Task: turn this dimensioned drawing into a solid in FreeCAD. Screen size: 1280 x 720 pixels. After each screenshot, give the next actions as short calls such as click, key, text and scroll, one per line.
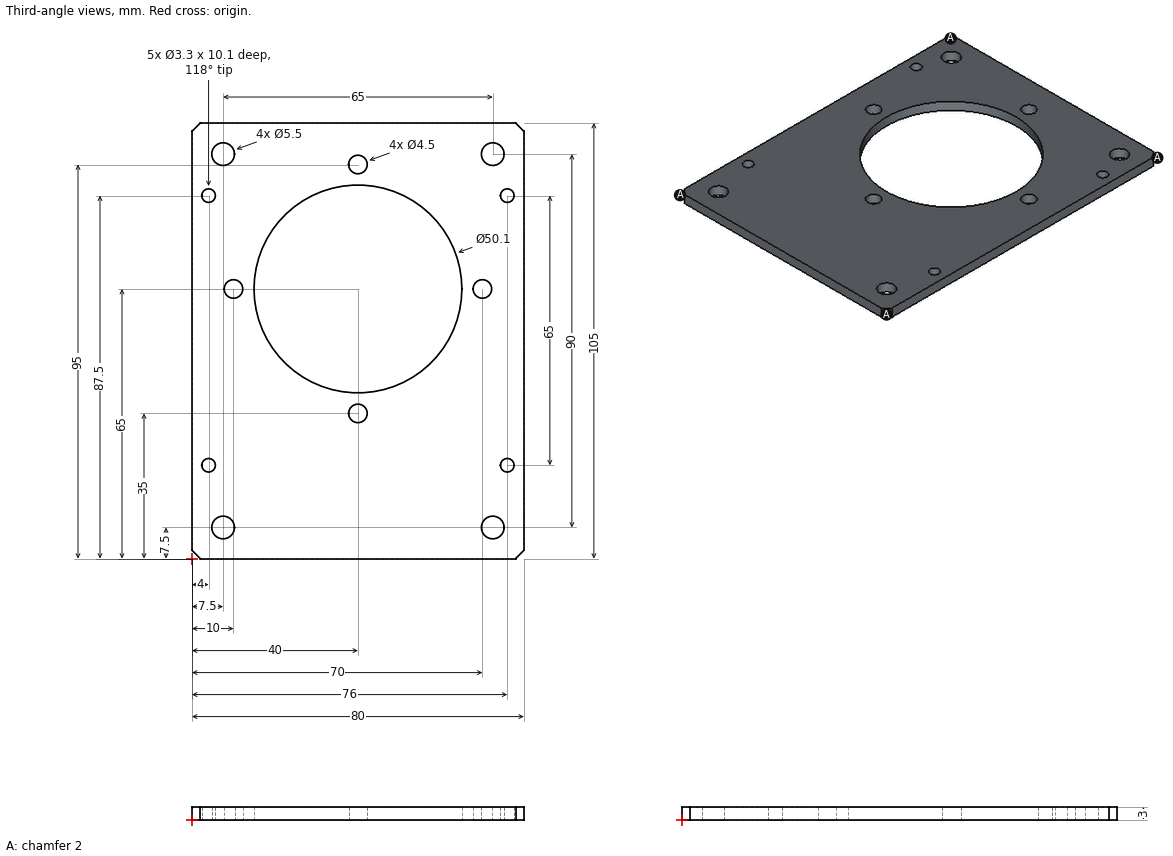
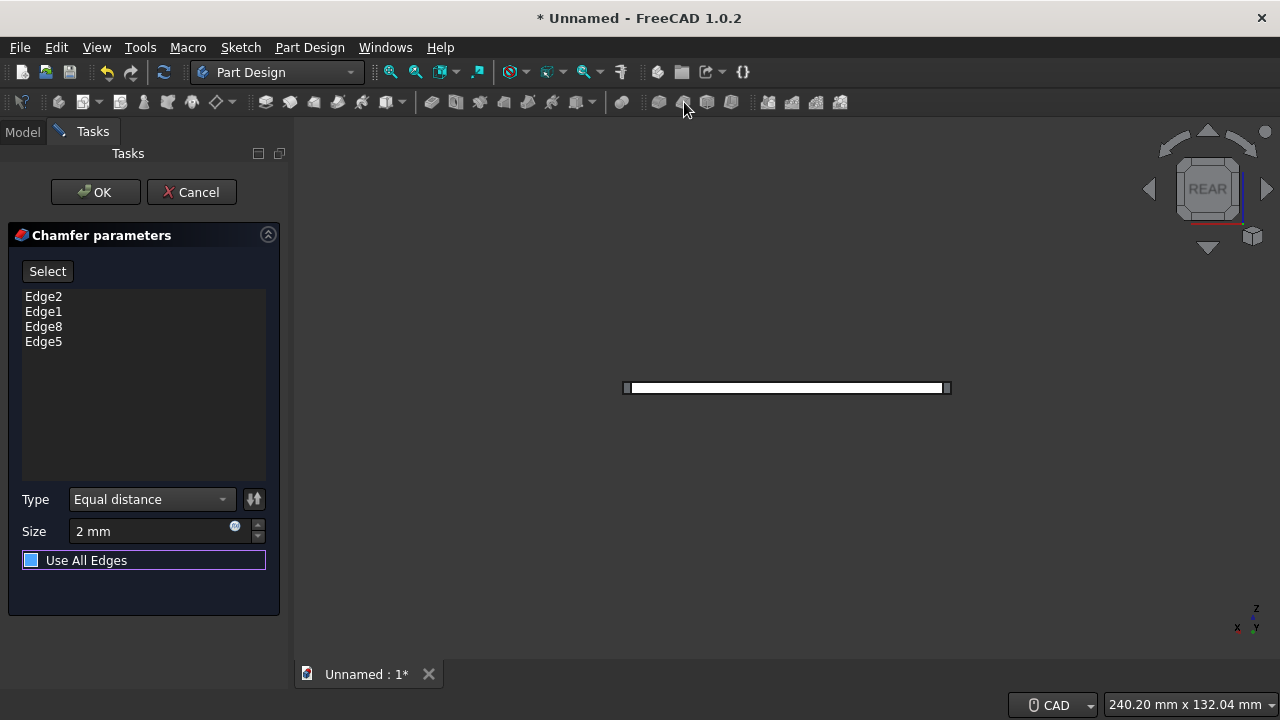
click(96, 192)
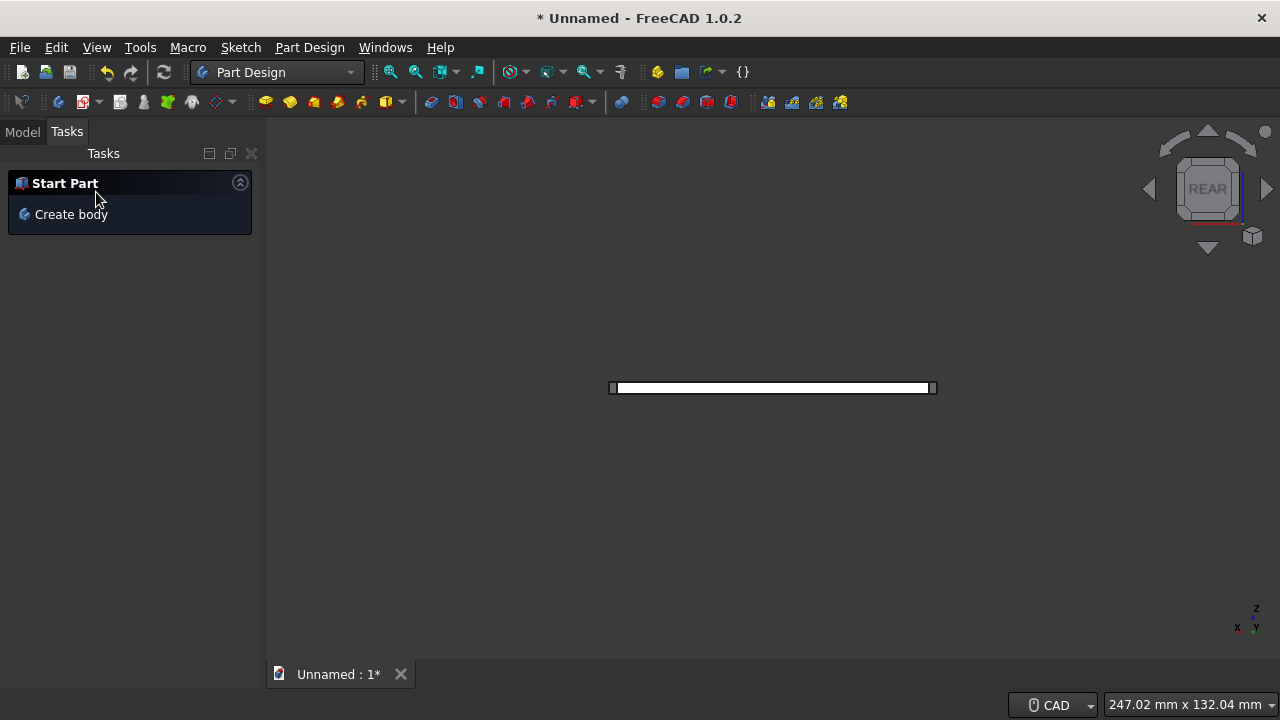
click(392, 72)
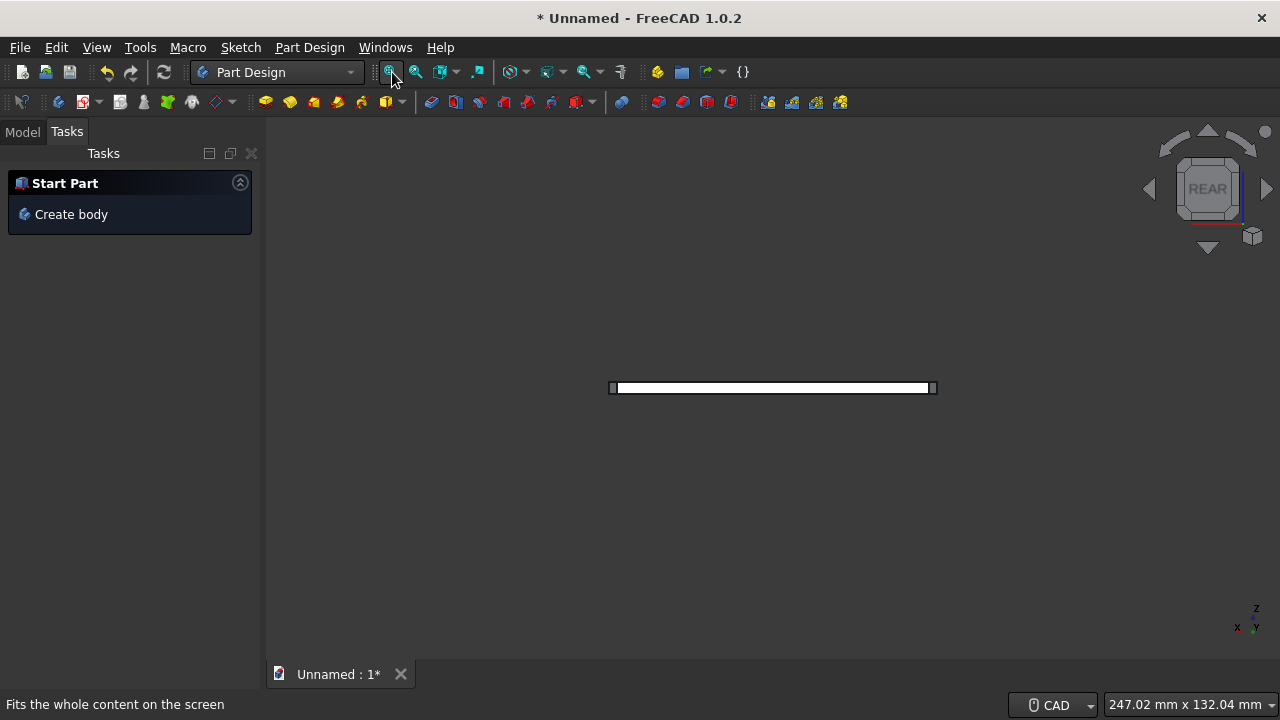
key(0)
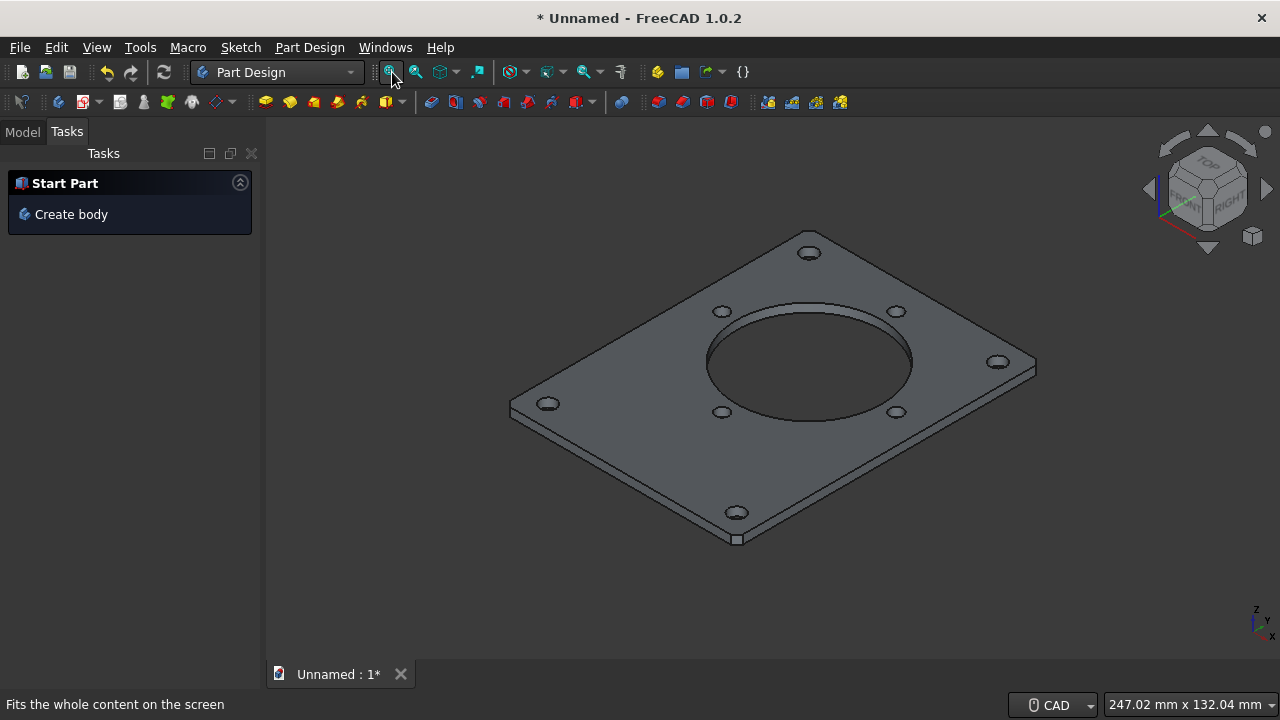
click(752, 471)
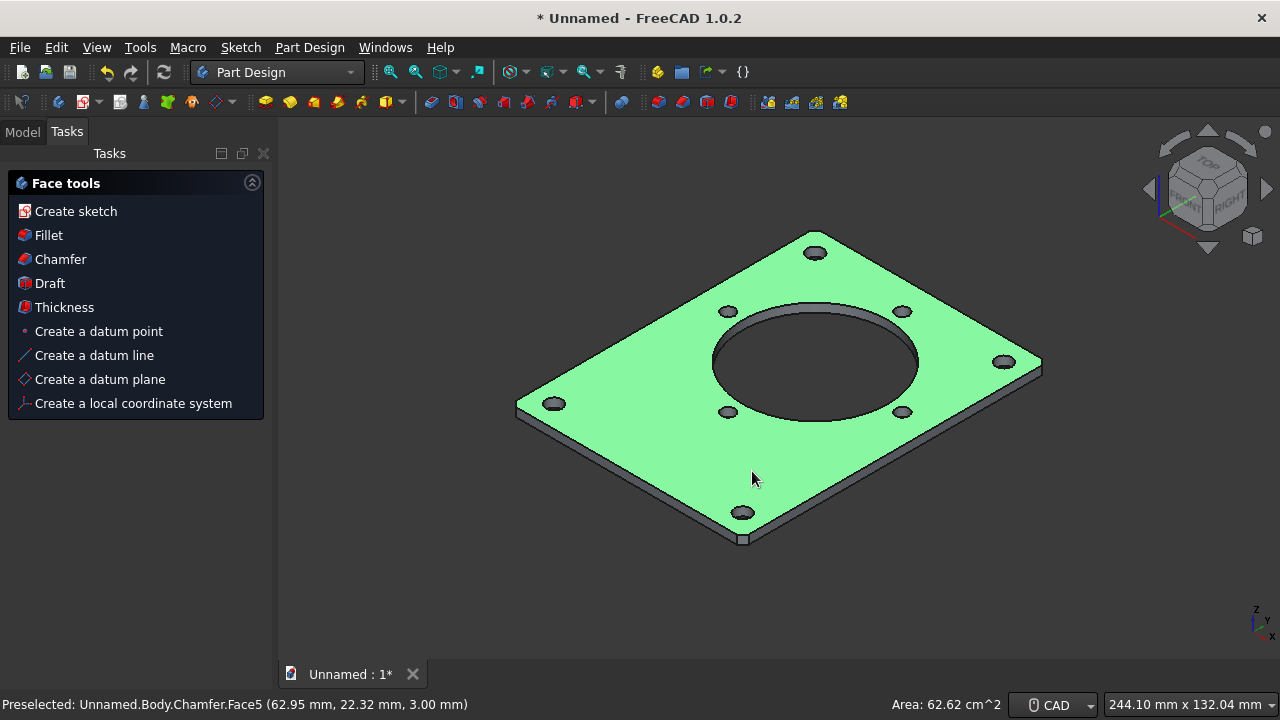
click(84, 102)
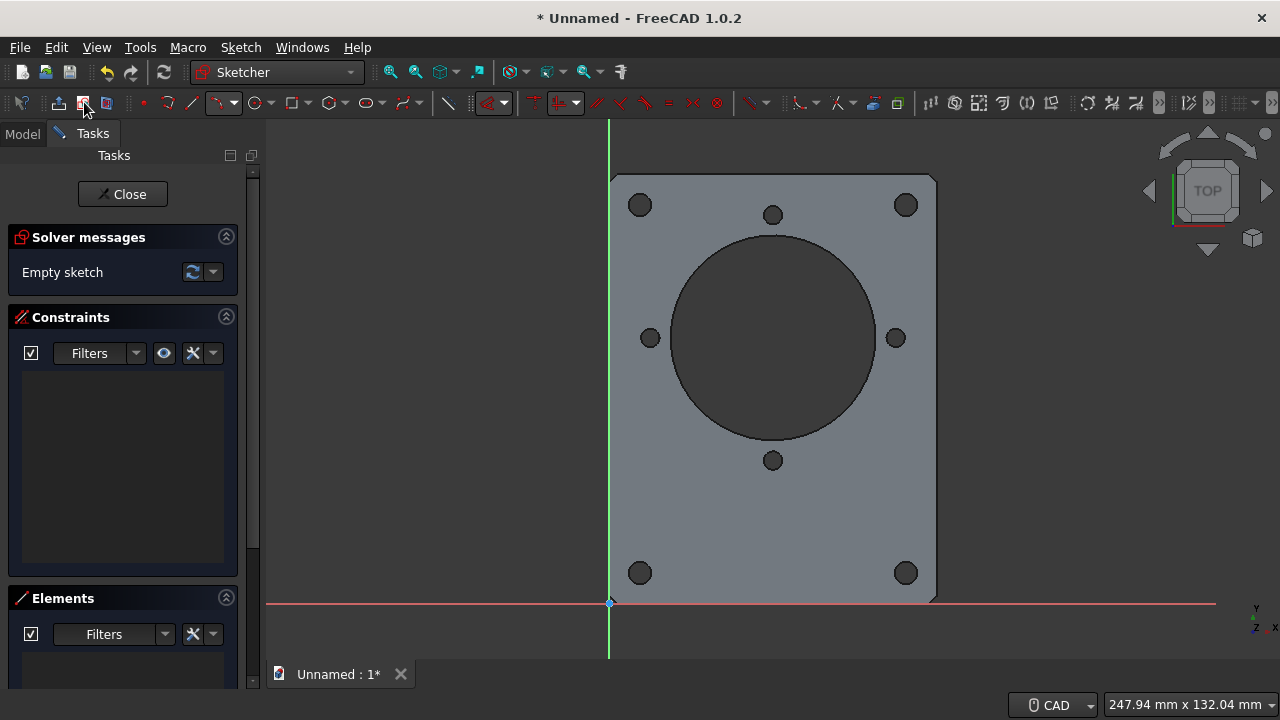
click(256, 104)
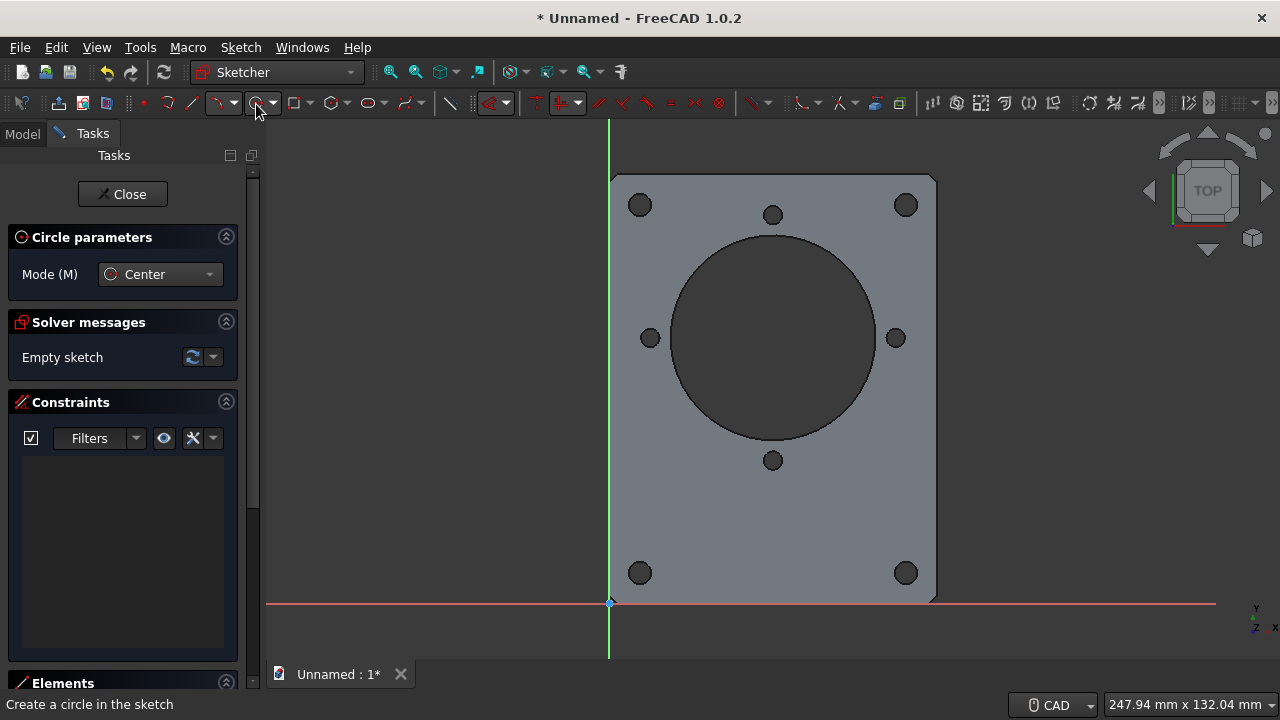
scroll(626, 246, up, 7)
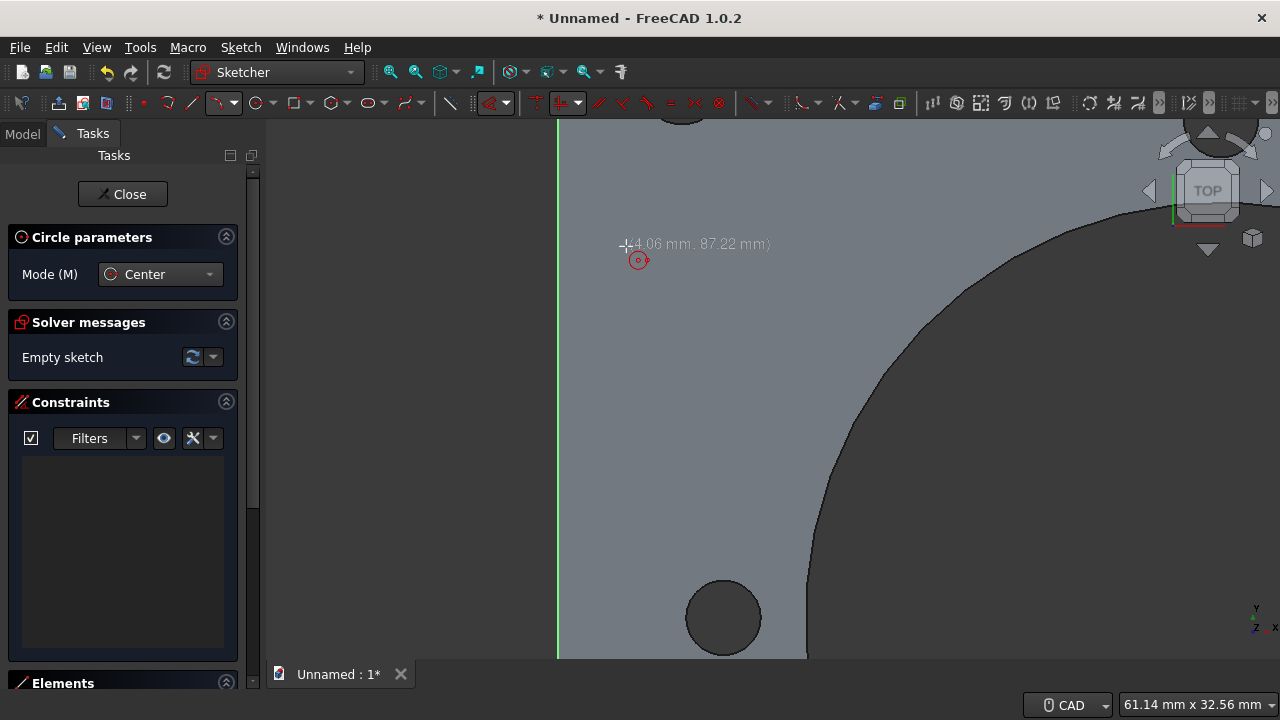
scroll(542, 203, down, 7)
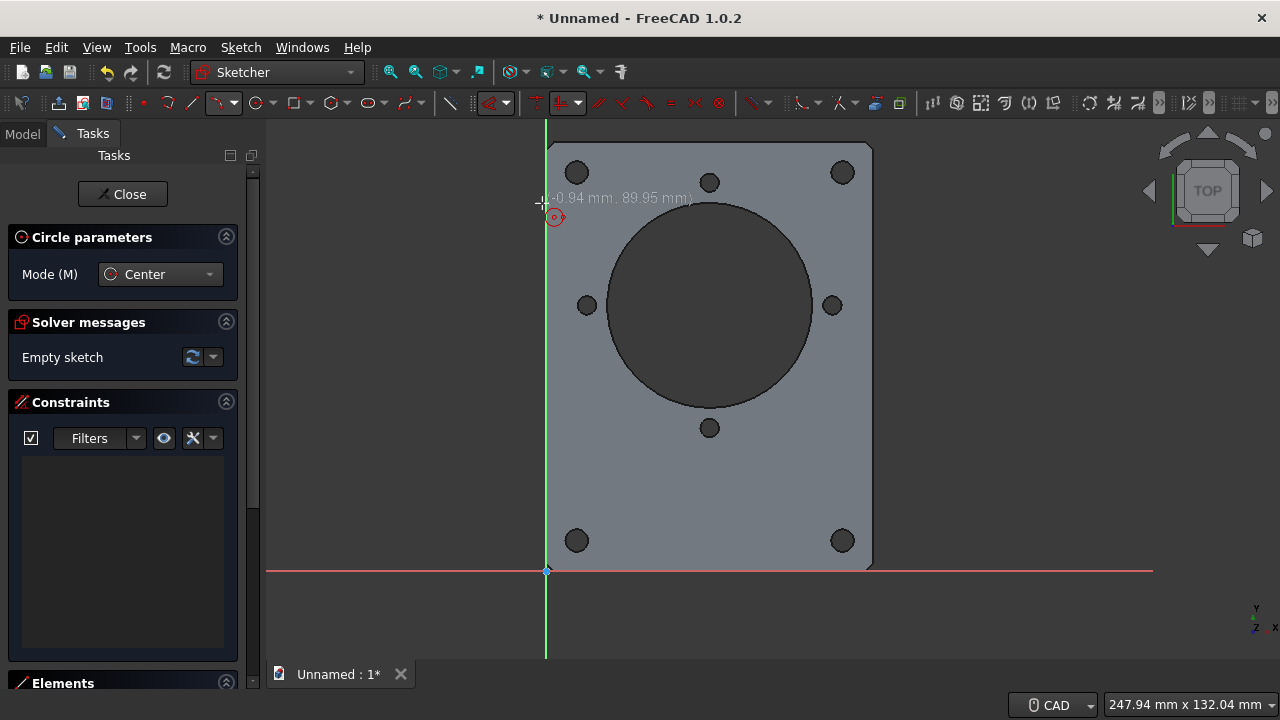
click(562, 213)
move(567, 209)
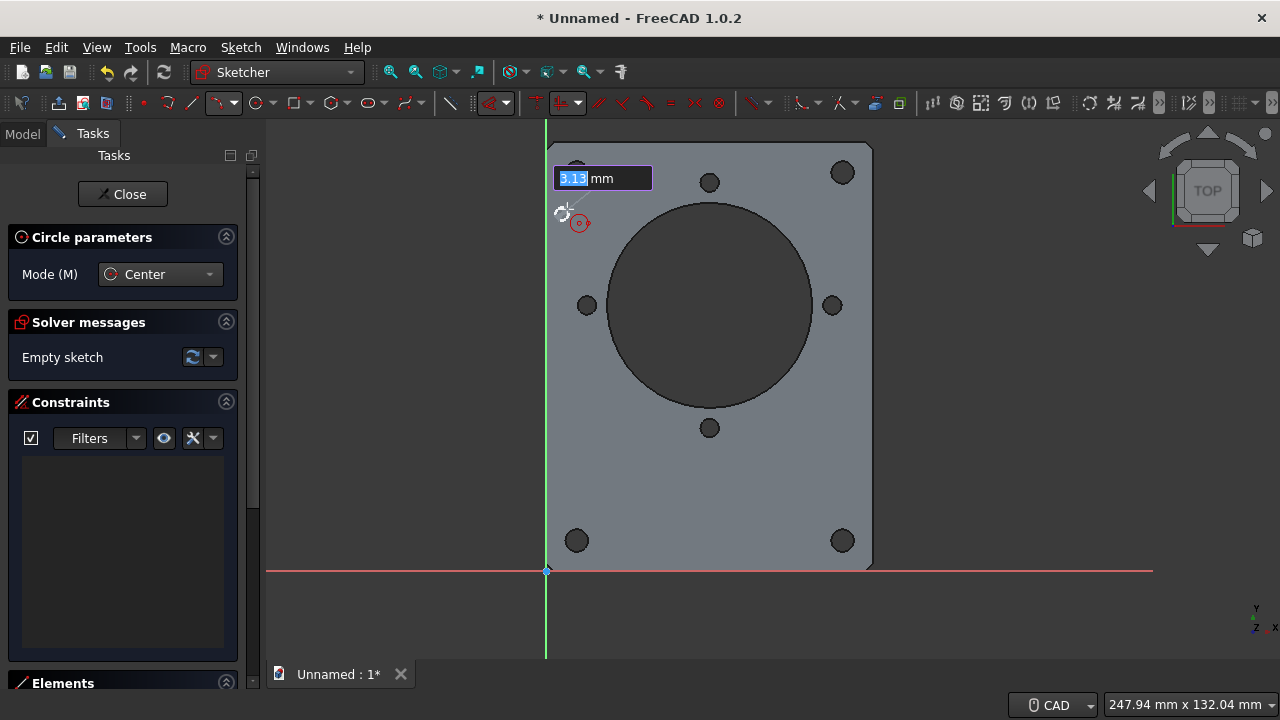
text(3.3)
key(Return)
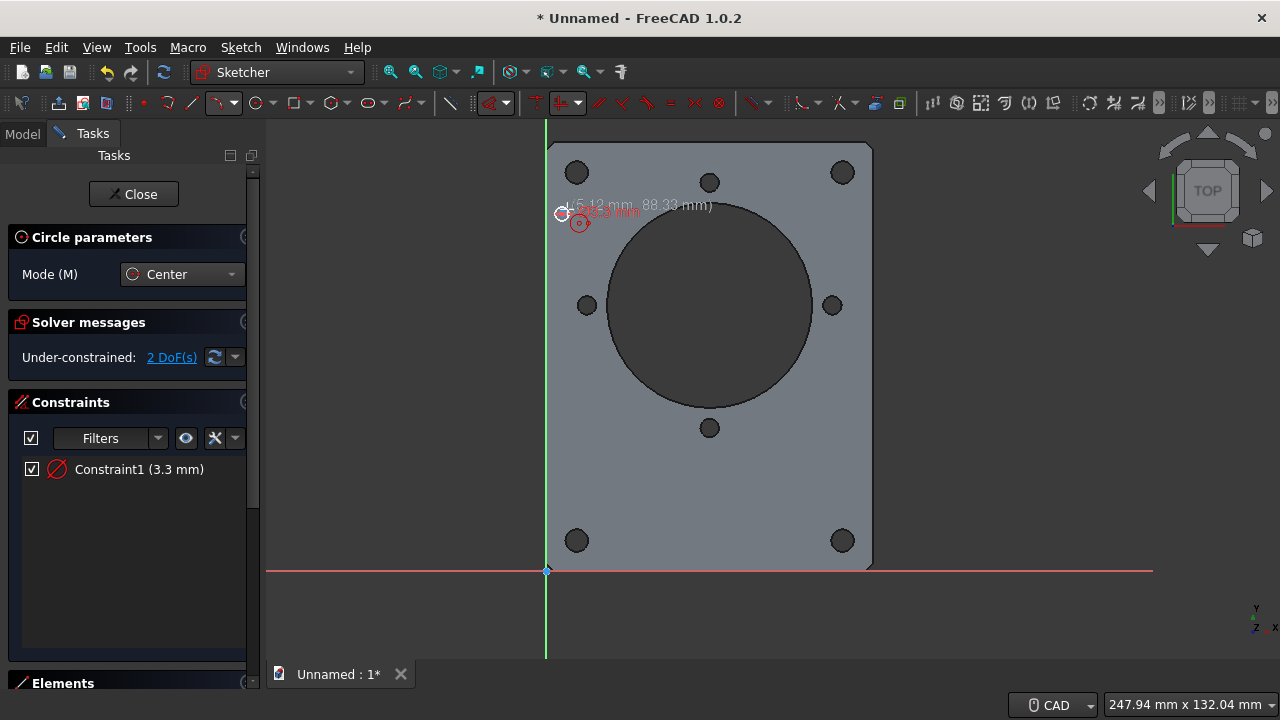
scroll(857, 213, up, 7)